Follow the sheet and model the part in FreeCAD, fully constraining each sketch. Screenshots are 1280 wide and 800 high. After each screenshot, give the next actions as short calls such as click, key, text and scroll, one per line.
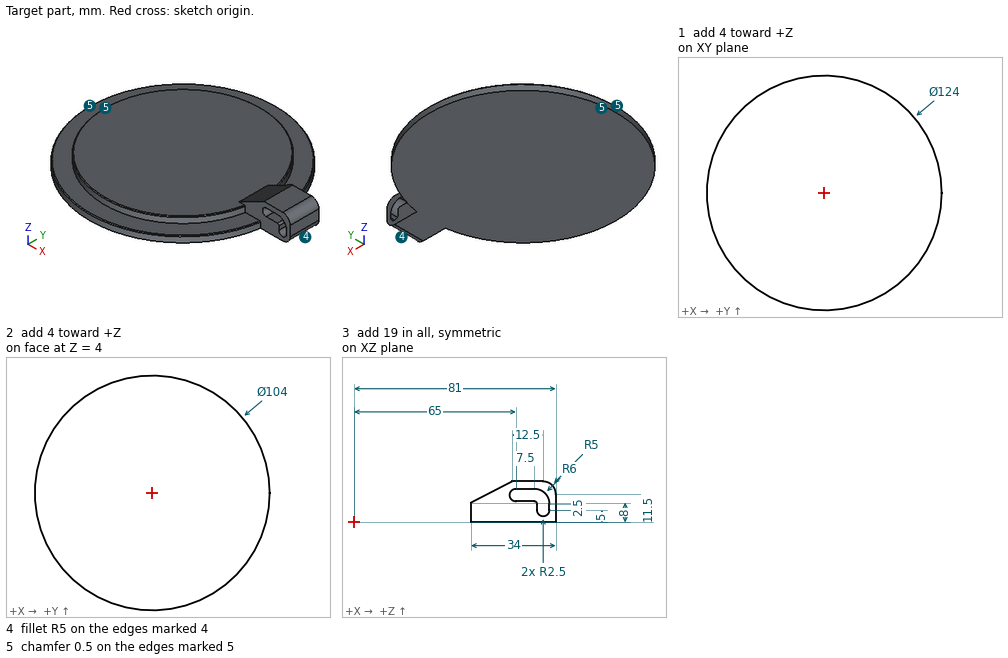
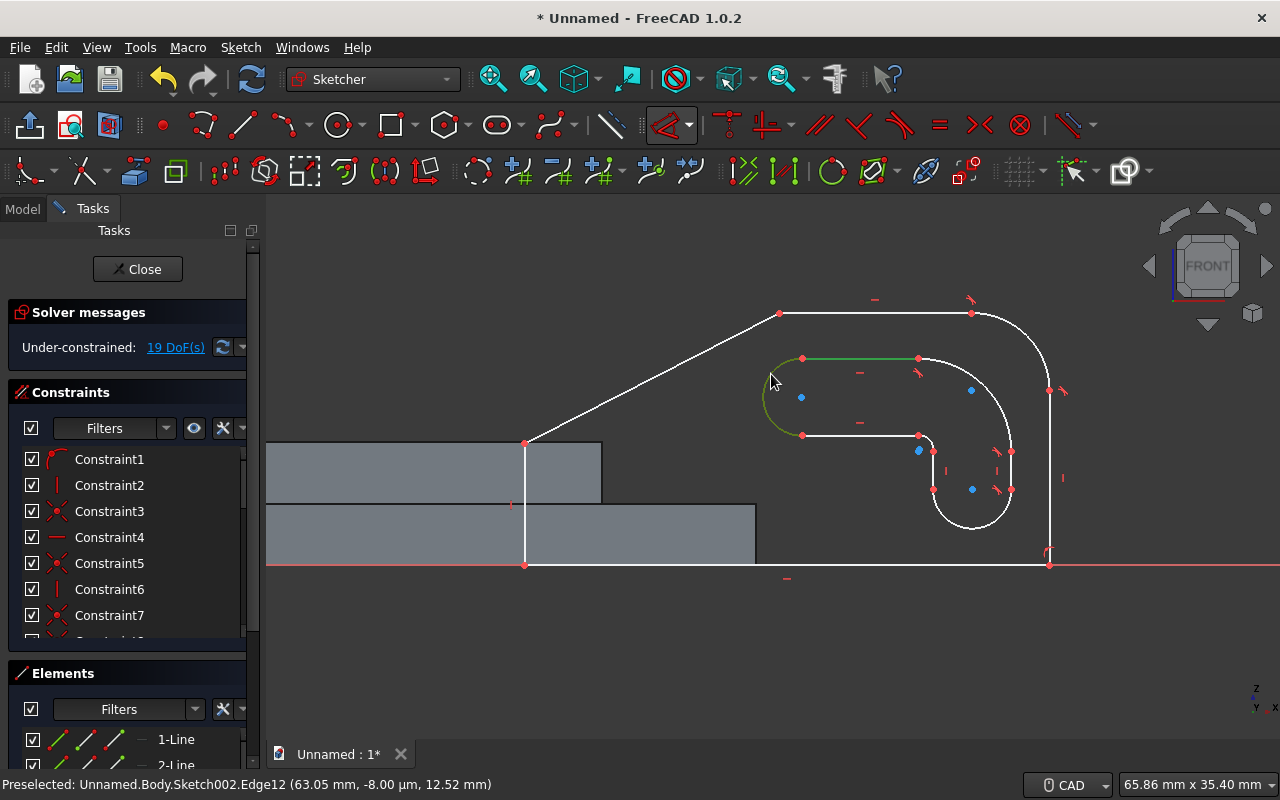
key(t)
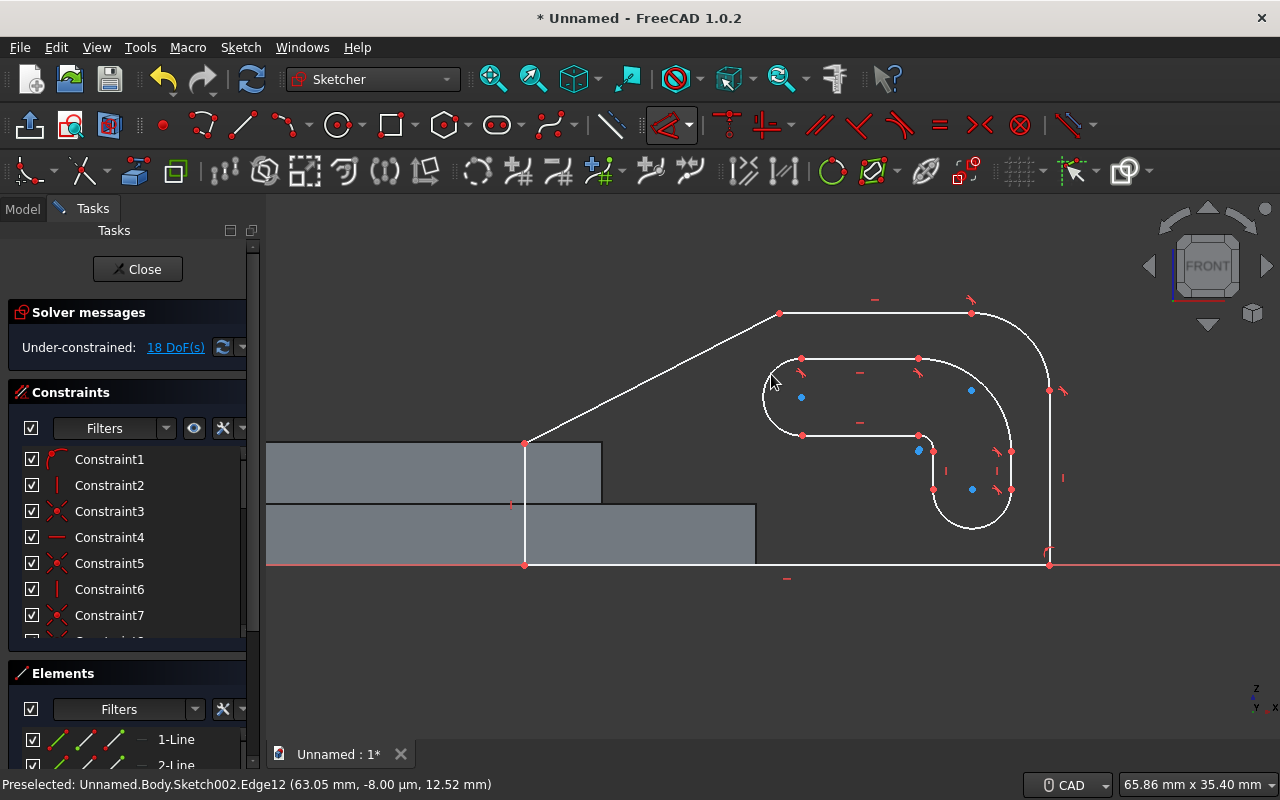
click(837, 436)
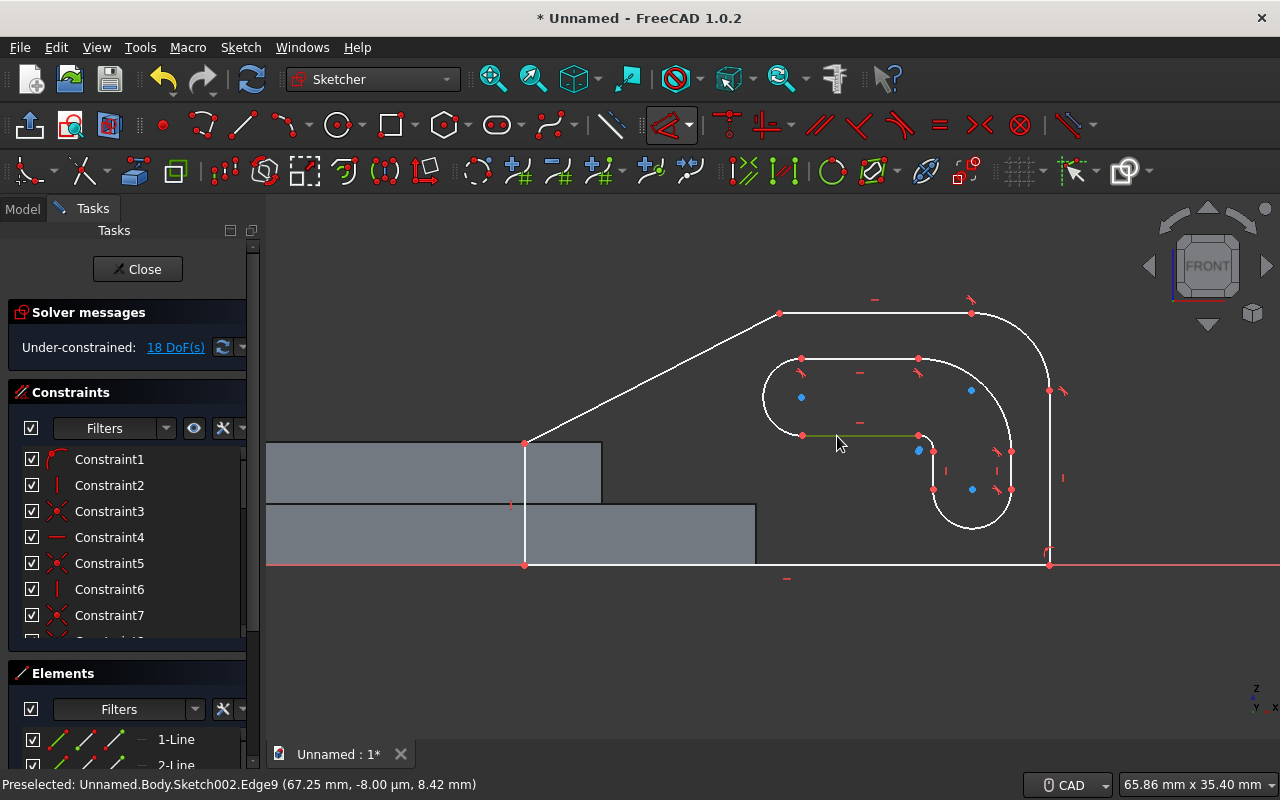
click(771, 375)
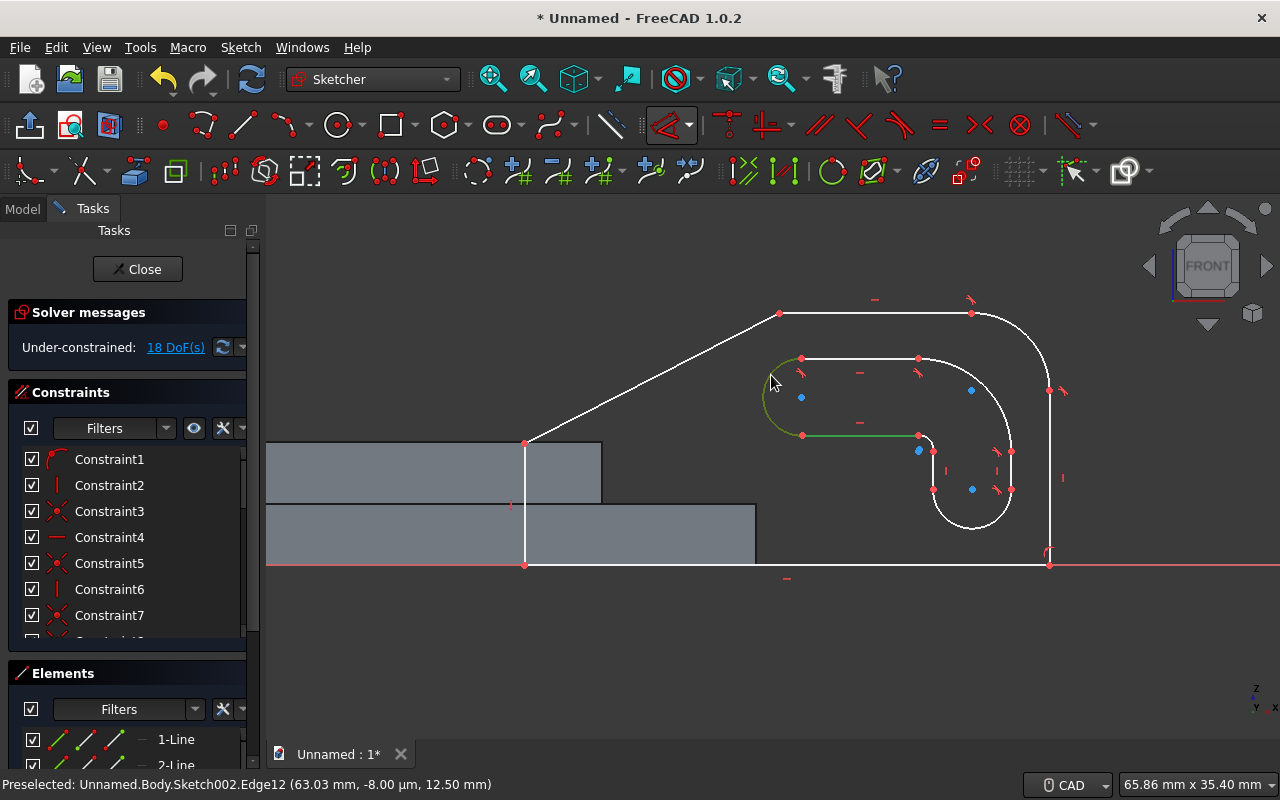
click(900, 126)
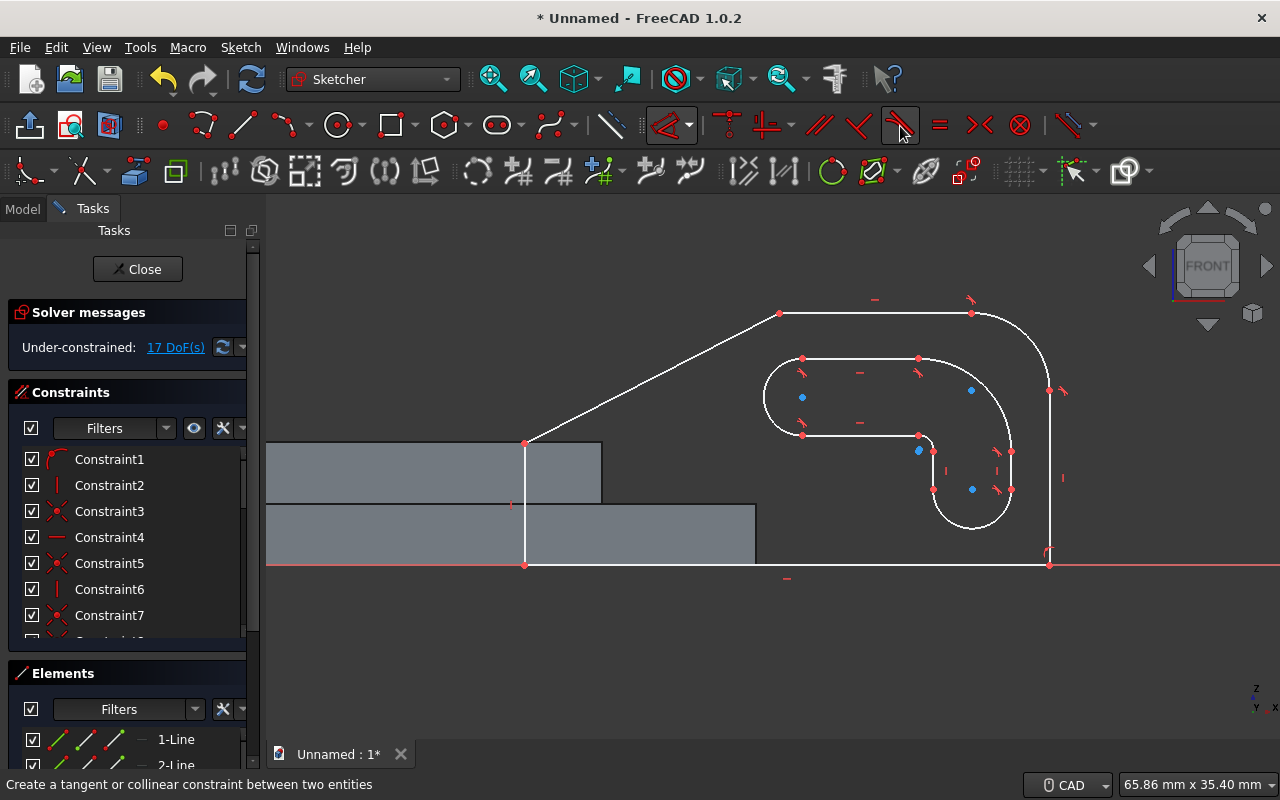
click(837, 436)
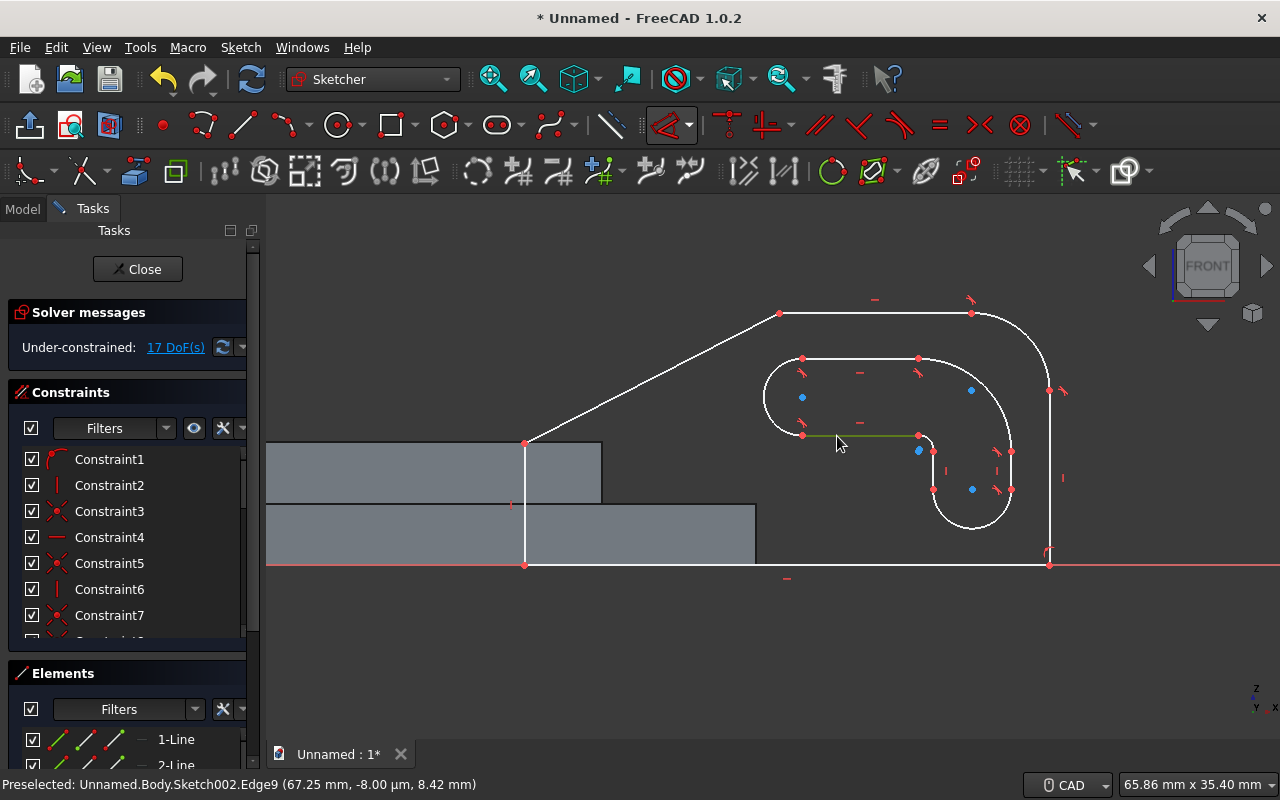
click(930, 440)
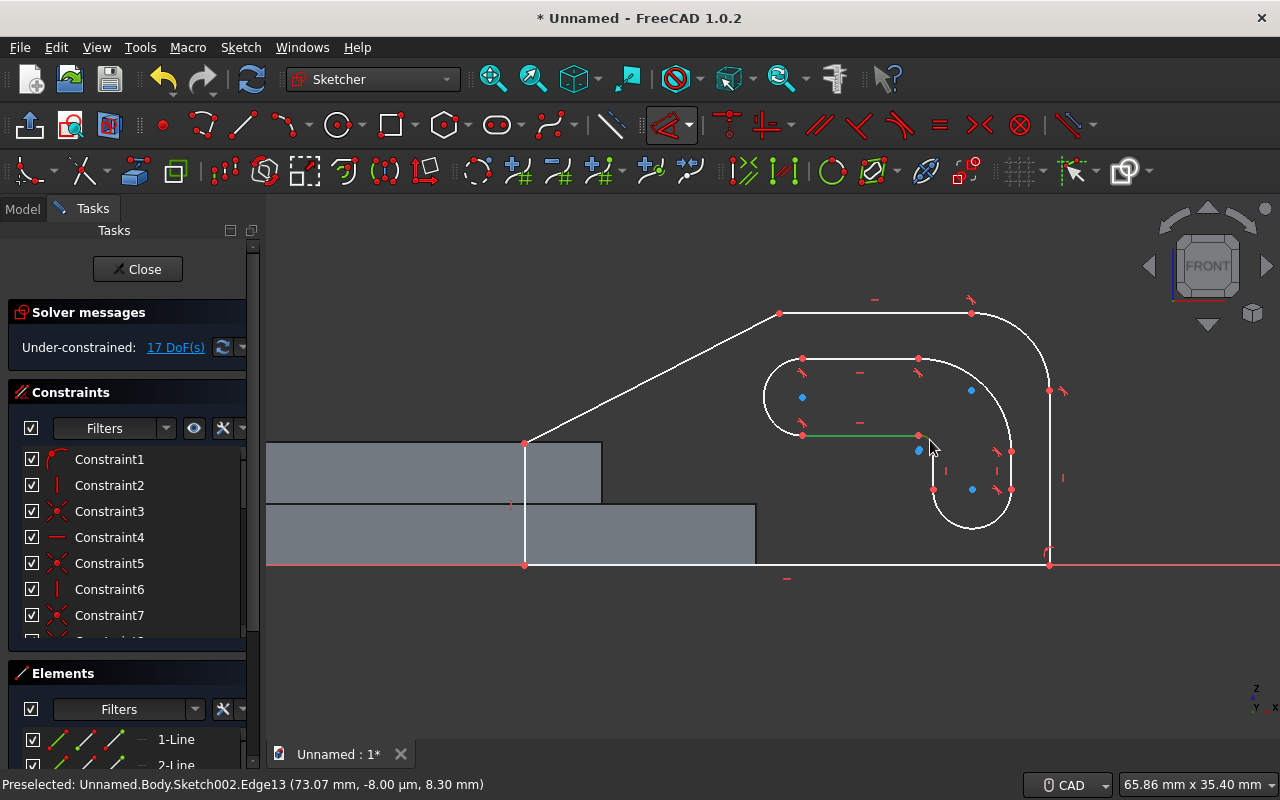
key(t)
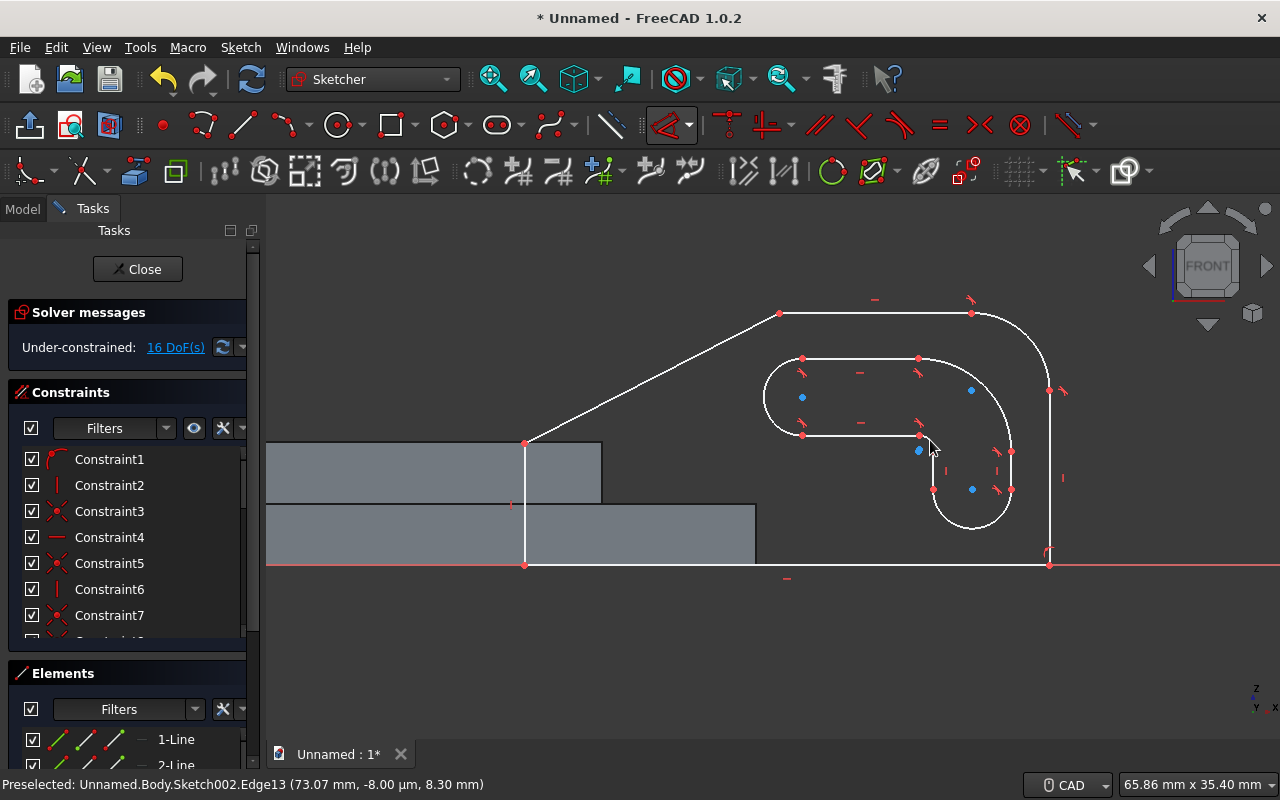
click(933, 463)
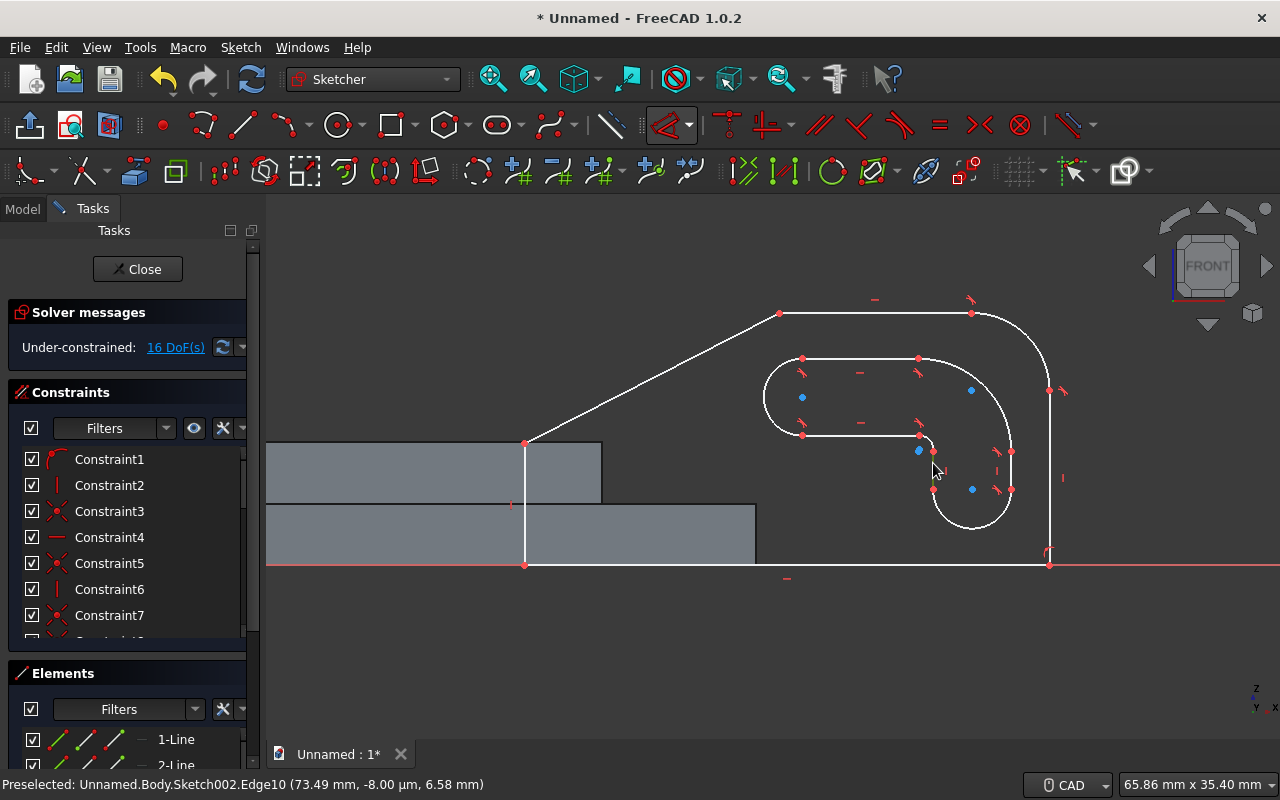
click(930, 441)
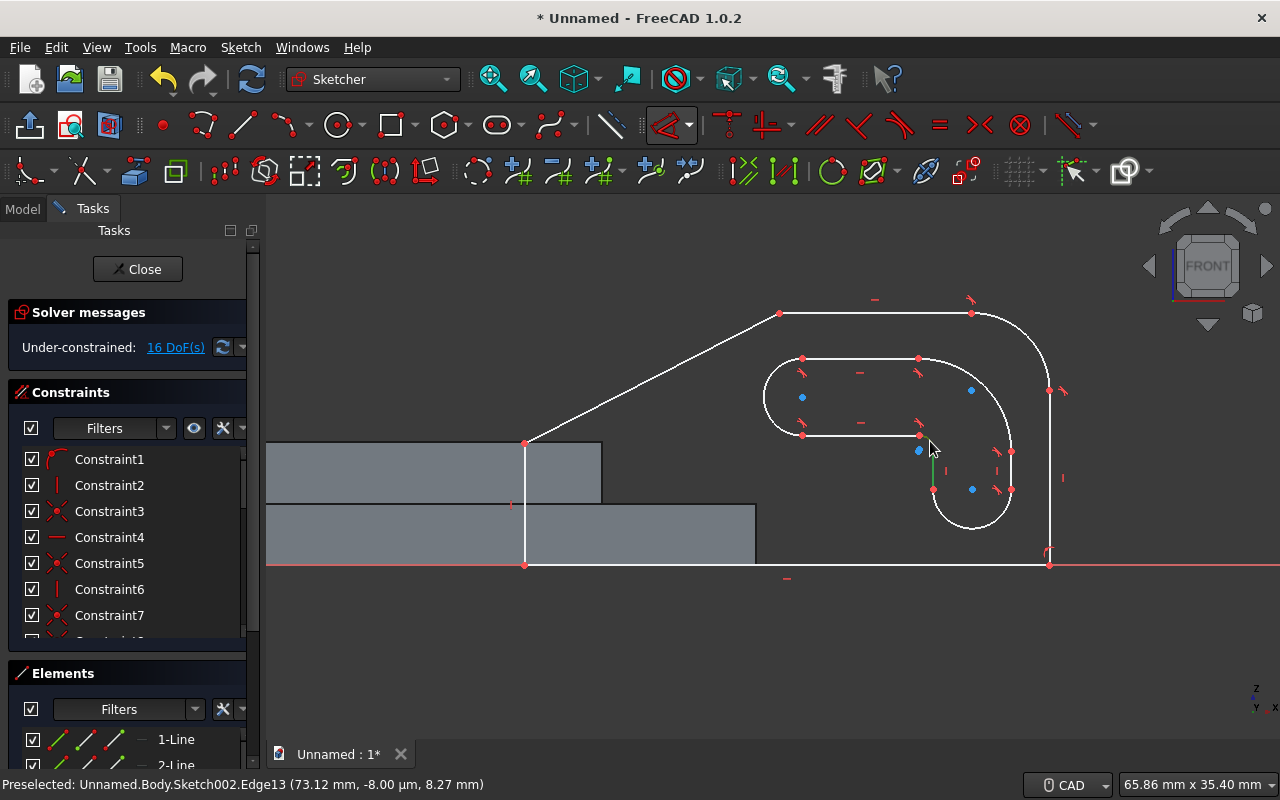
click(900, 126)